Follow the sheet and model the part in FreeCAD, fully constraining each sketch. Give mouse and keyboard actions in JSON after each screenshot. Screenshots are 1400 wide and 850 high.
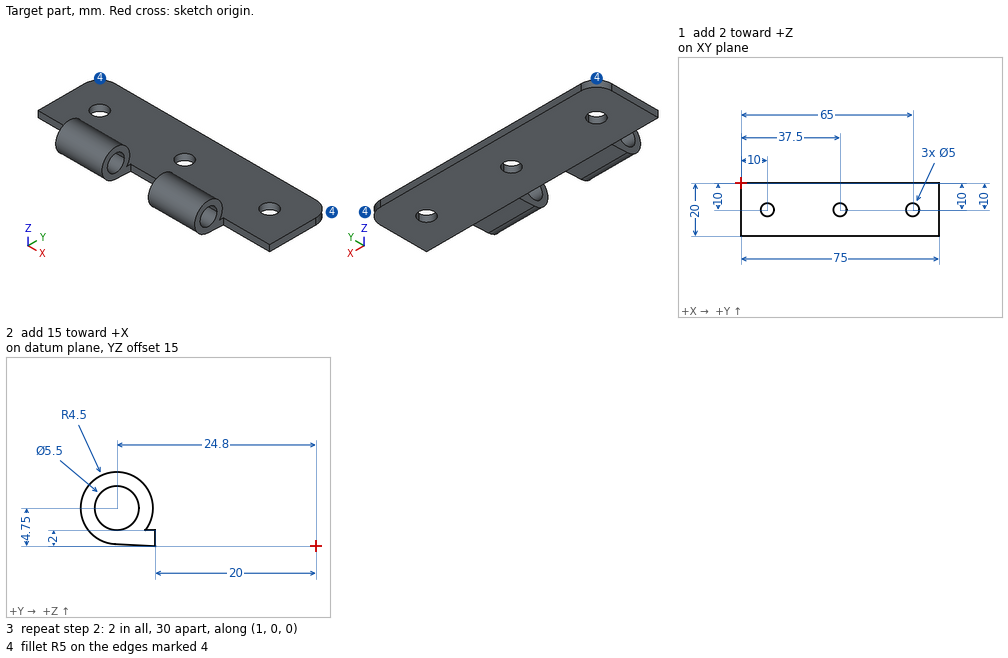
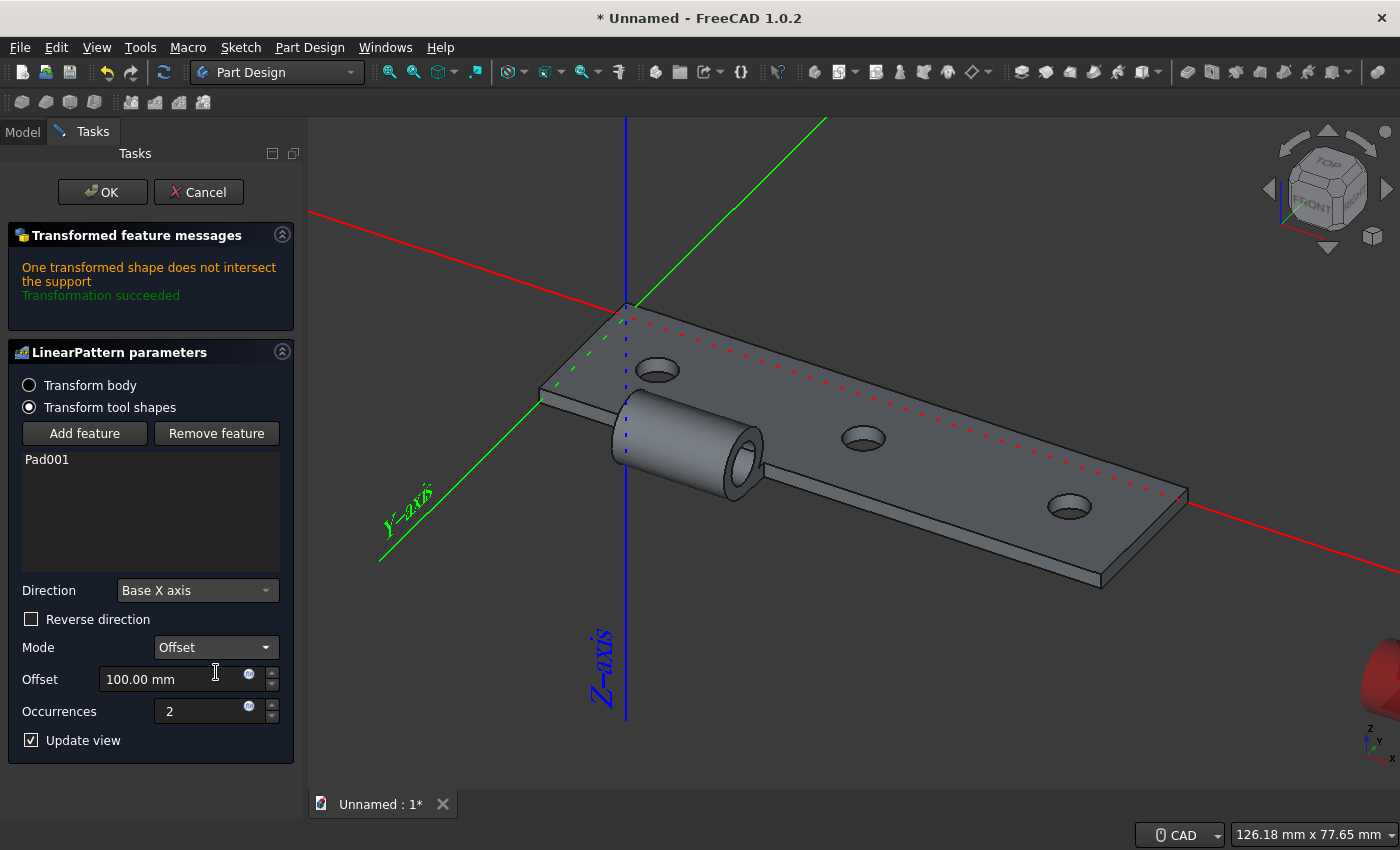
{"action": "triple_click", "coordinate": [182, 679]}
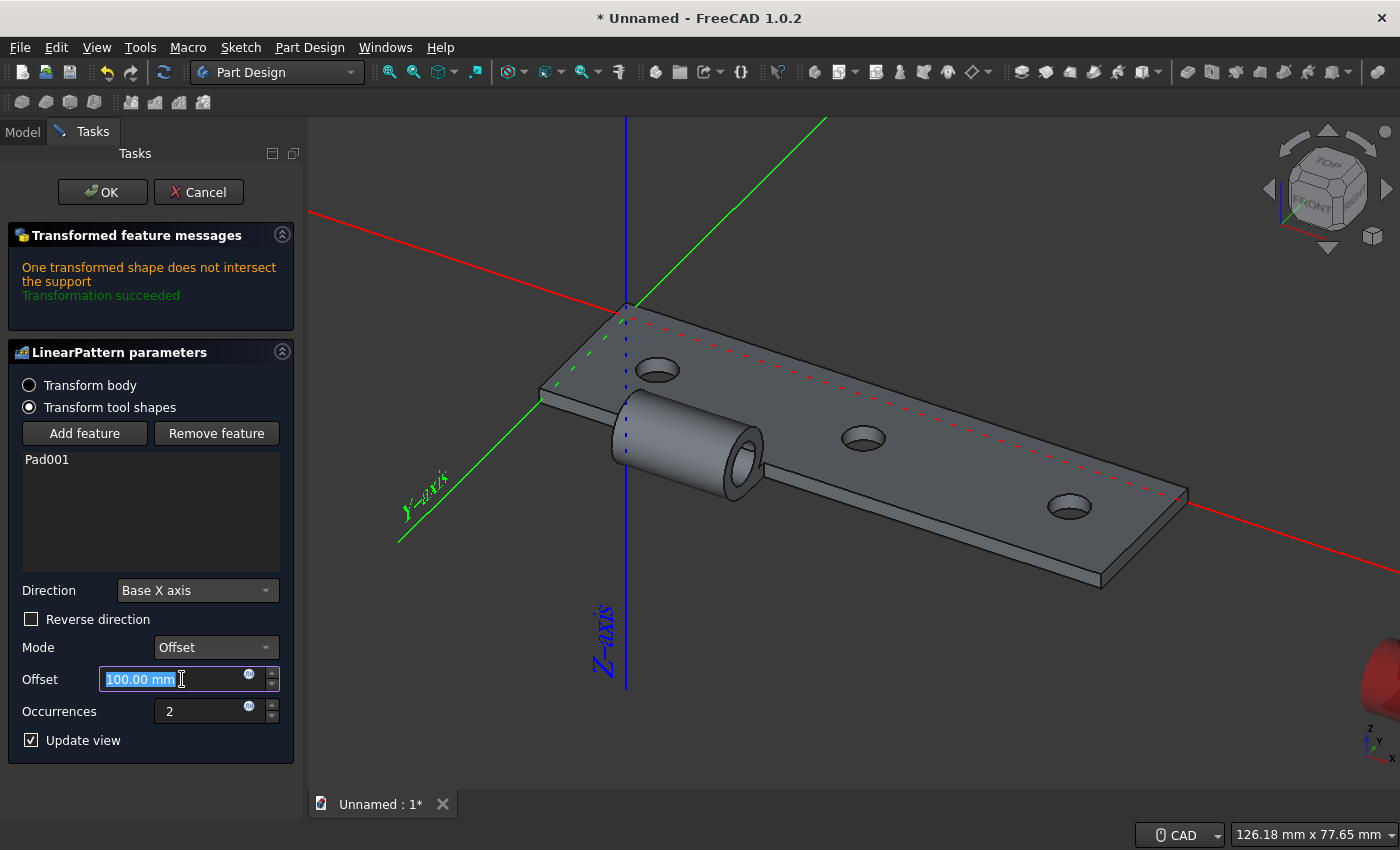
{"action": "type", "text": "30"}
{"action": "key", "text": "Tab"}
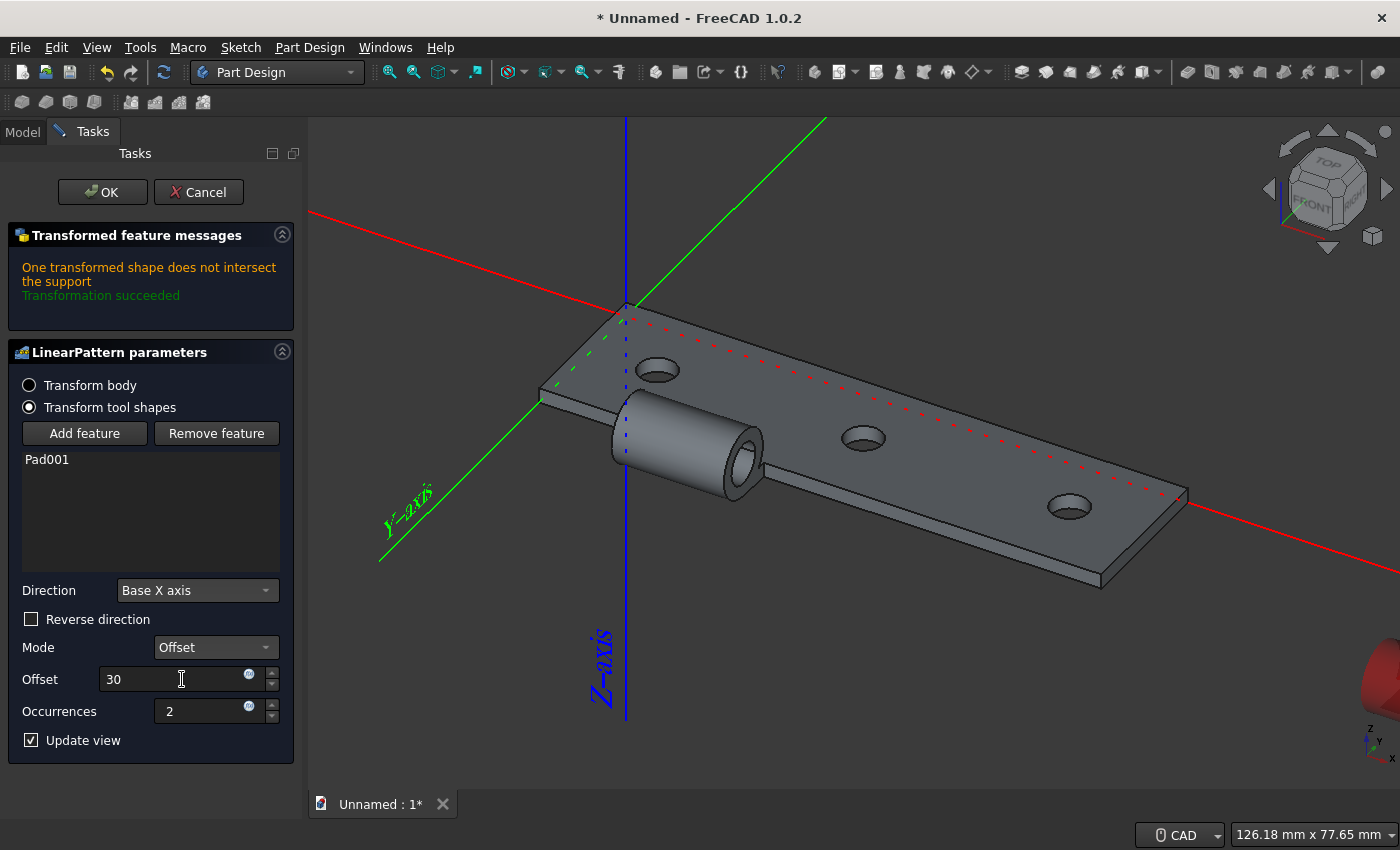
{"action": "triple_click", "coordinate": [209, 711]}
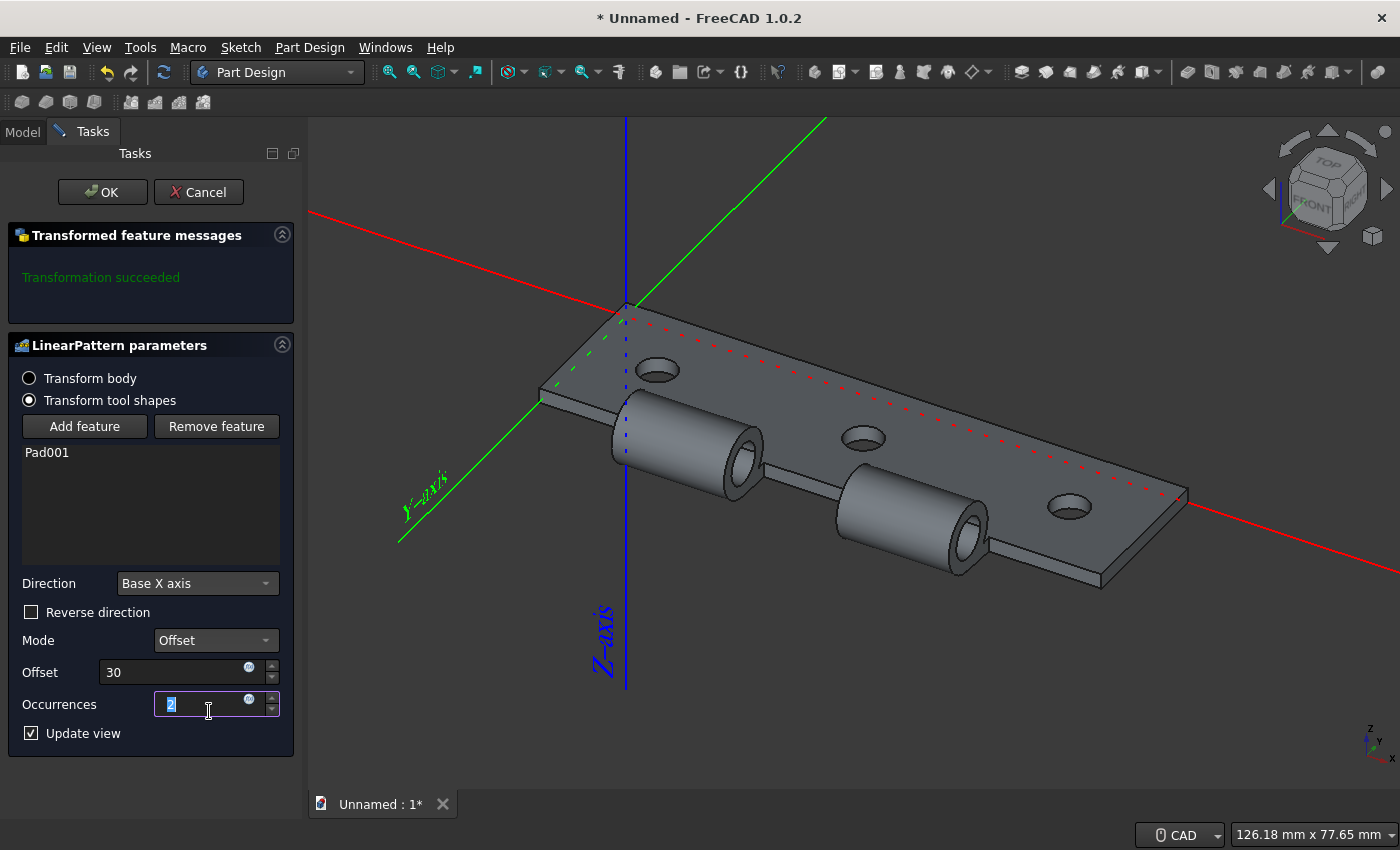
{"action": "type", "text": "2"}
{"action": "key", "text": "Tab"}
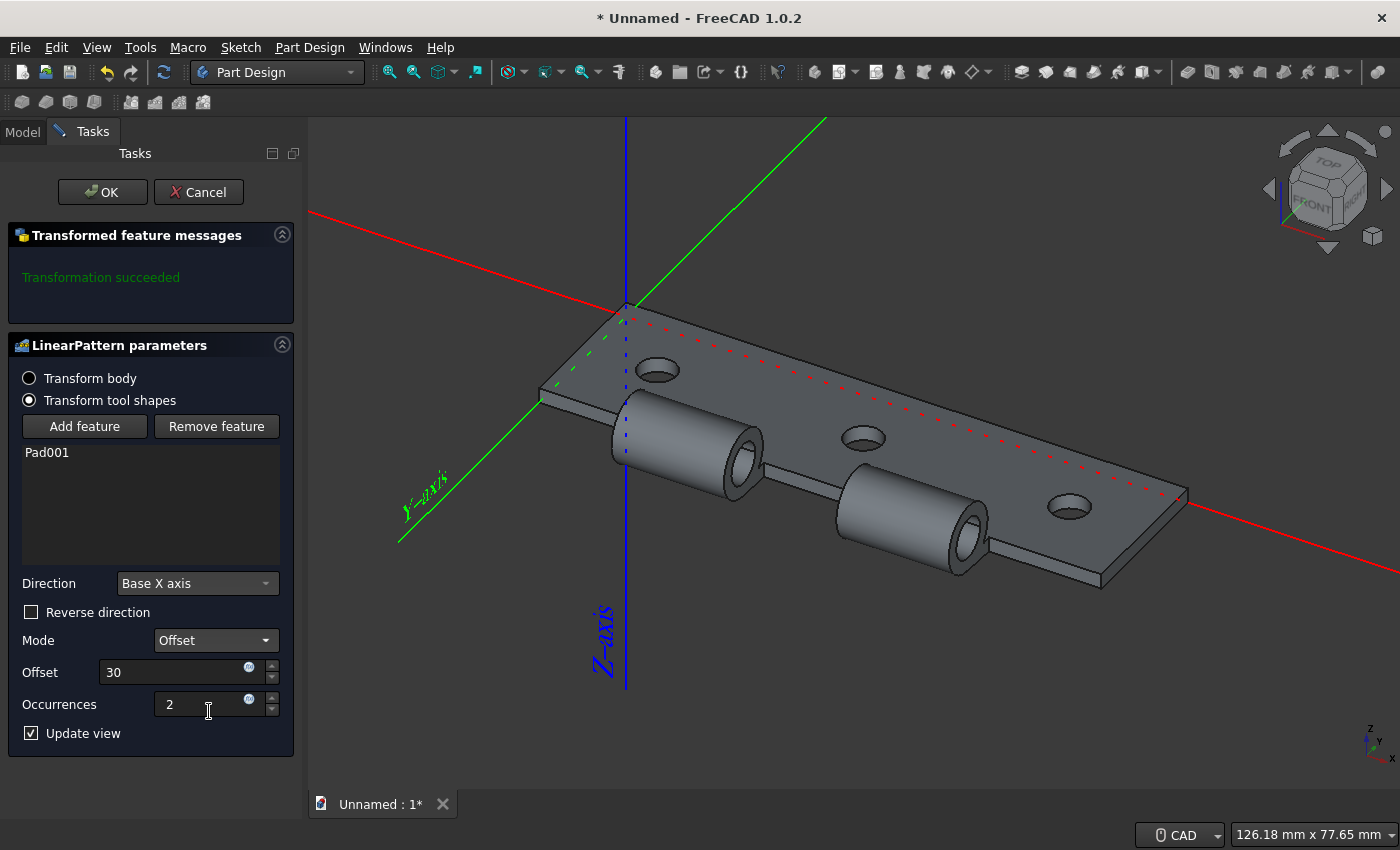
{"action": "left_click", "coordinate": [103, 192]}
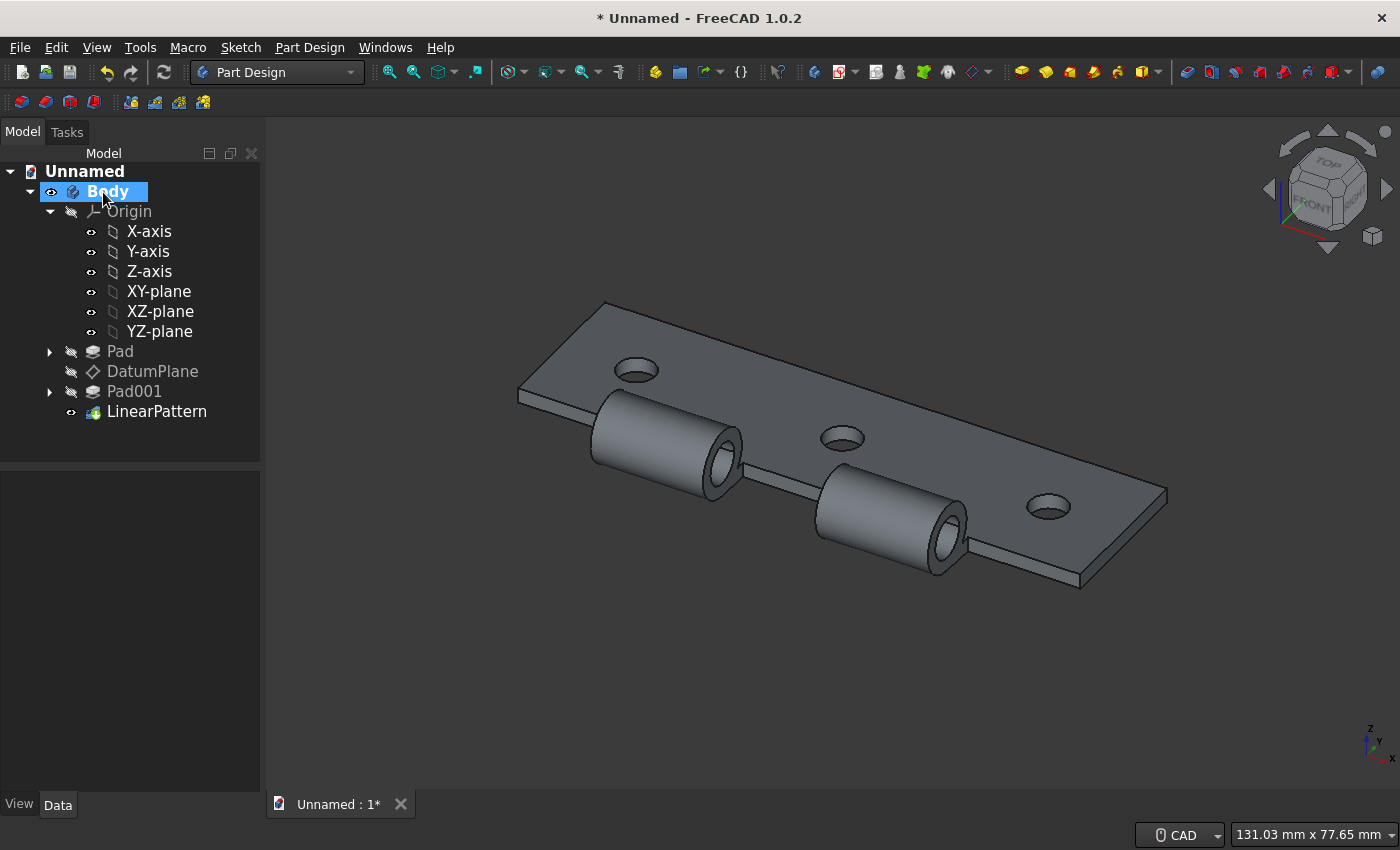
{"action": "scroll", "coordinate": [605, 308], "scroll_direction": "up", "scroll_amount": 5}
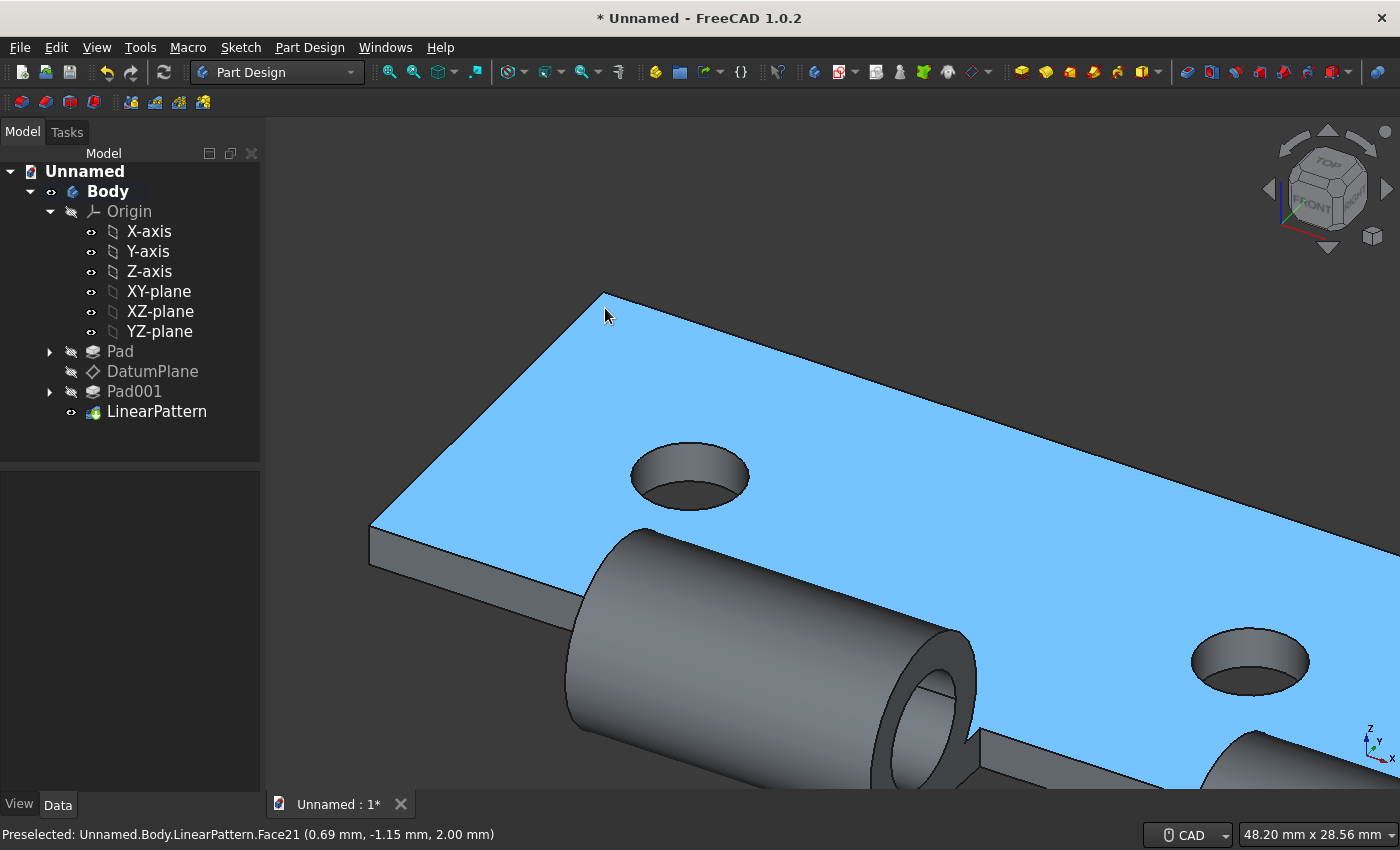
{"action": "key", "text": "v f"}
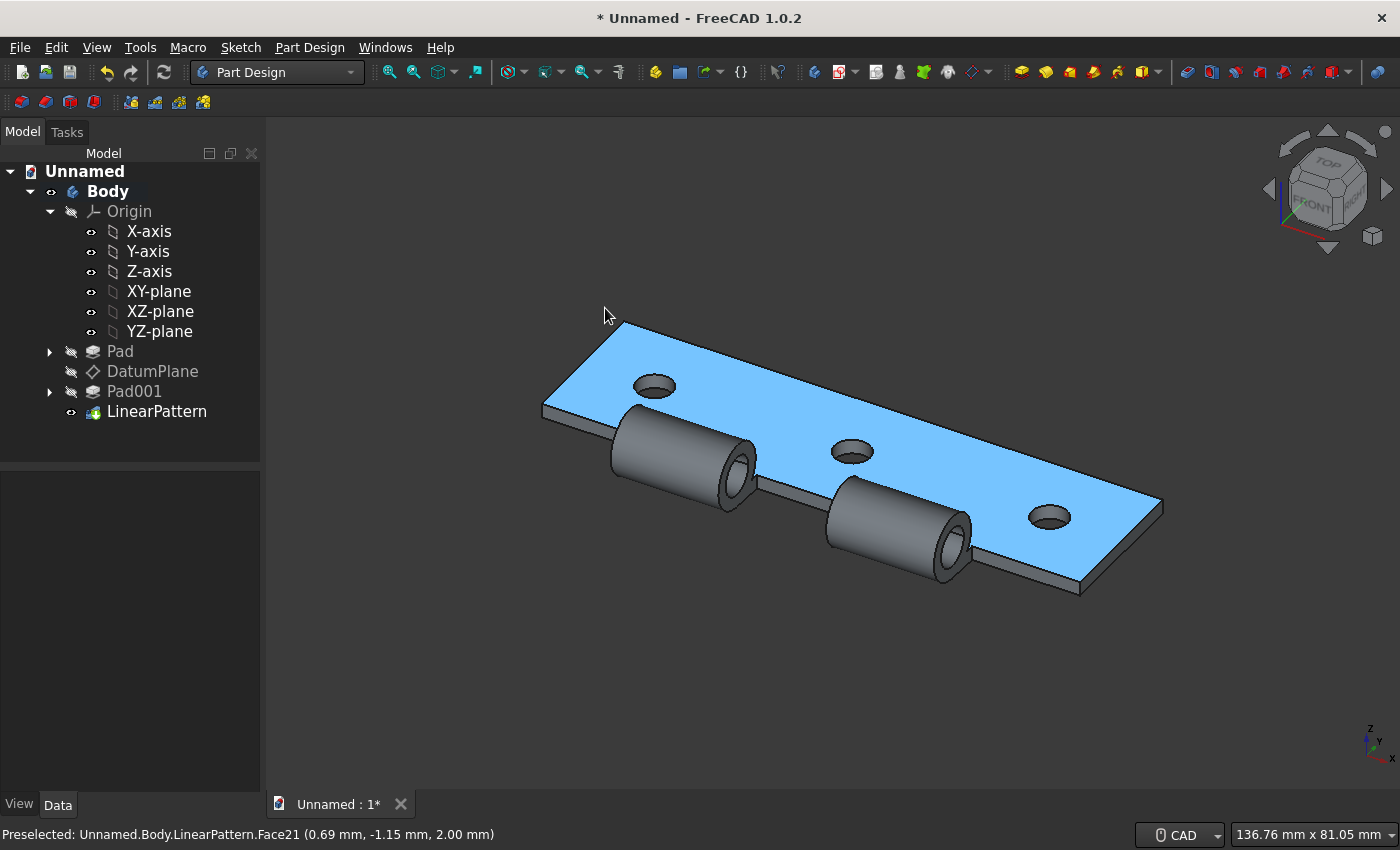
{"action": "key", "text": "0"}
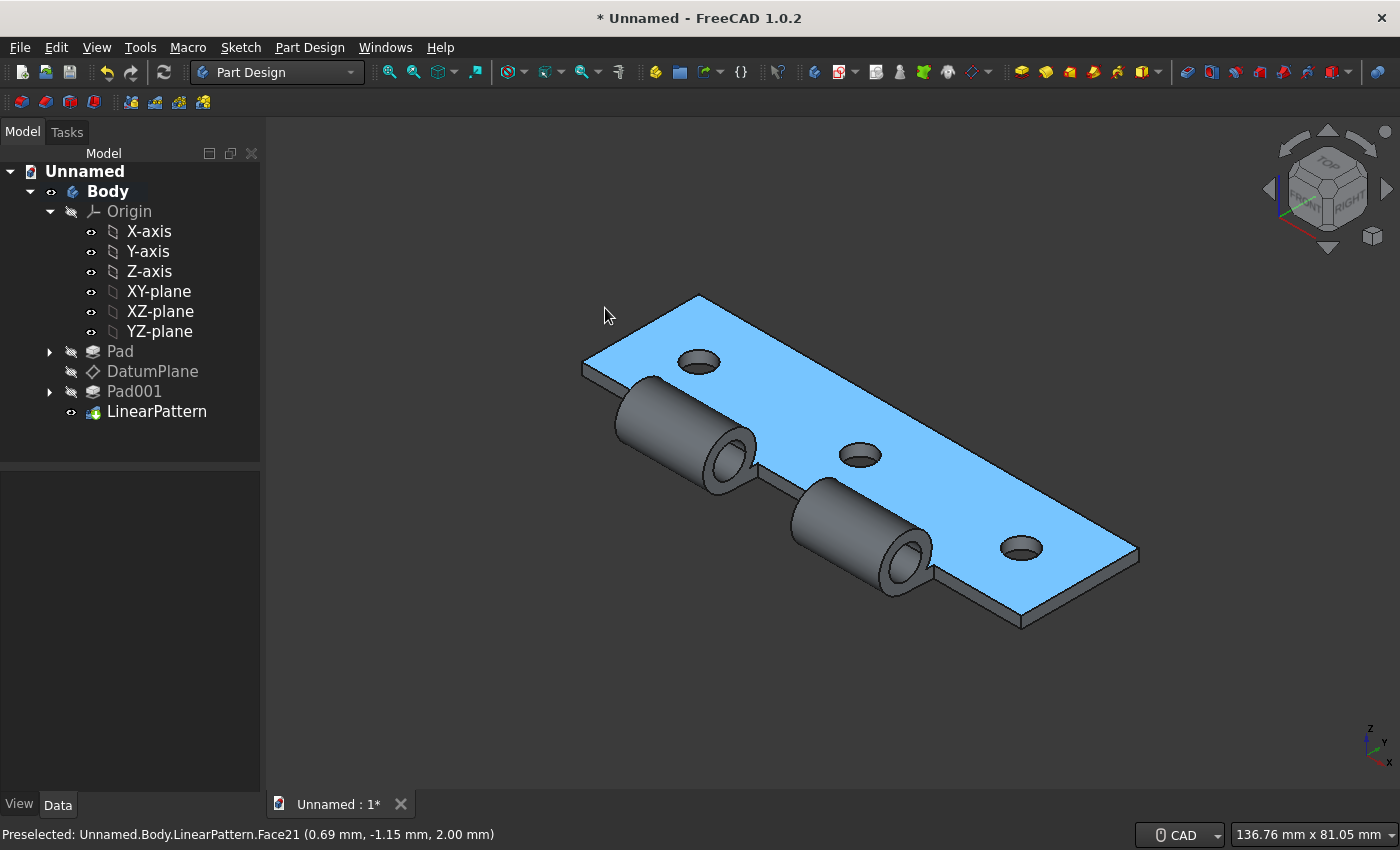
{"action": "scroll", "coordinate": [699, 300], "scroll_direction": "up", "scroll_amount": 5}